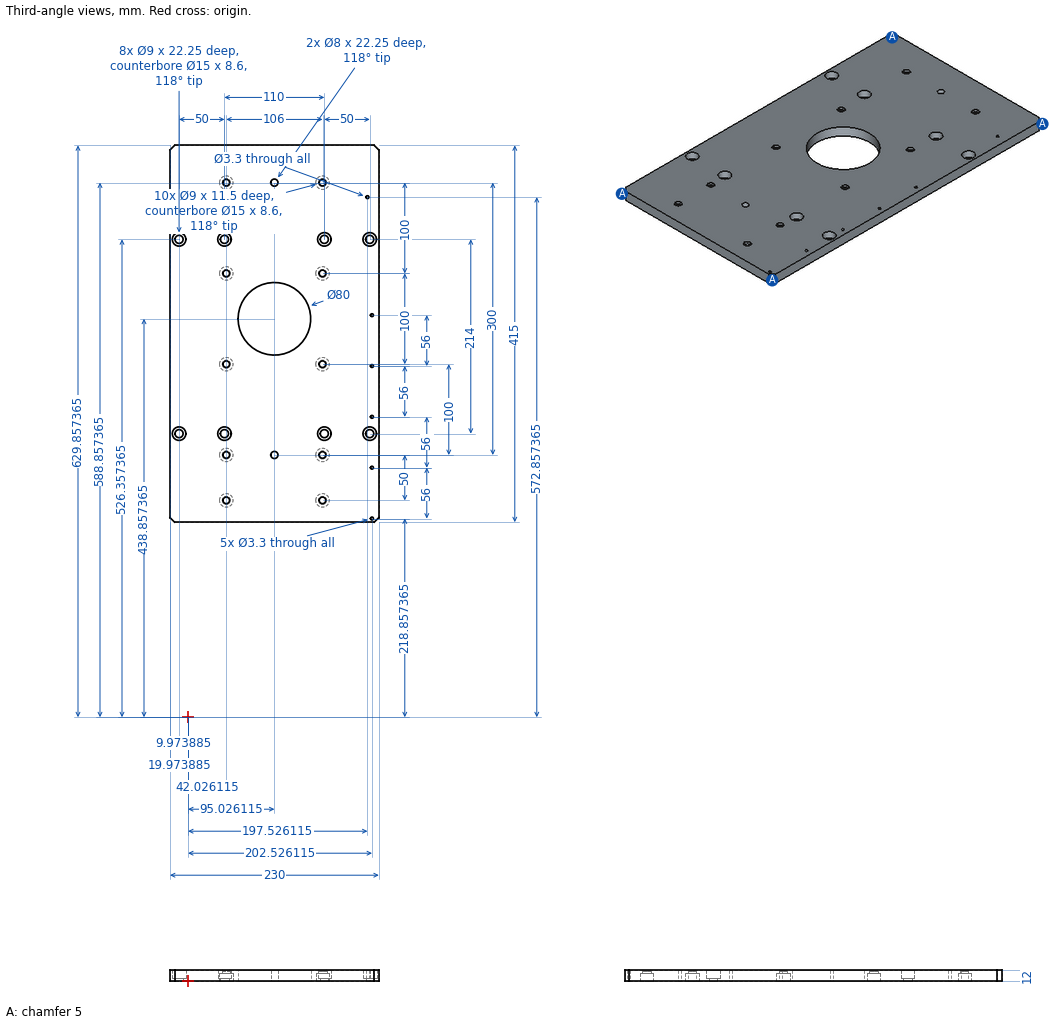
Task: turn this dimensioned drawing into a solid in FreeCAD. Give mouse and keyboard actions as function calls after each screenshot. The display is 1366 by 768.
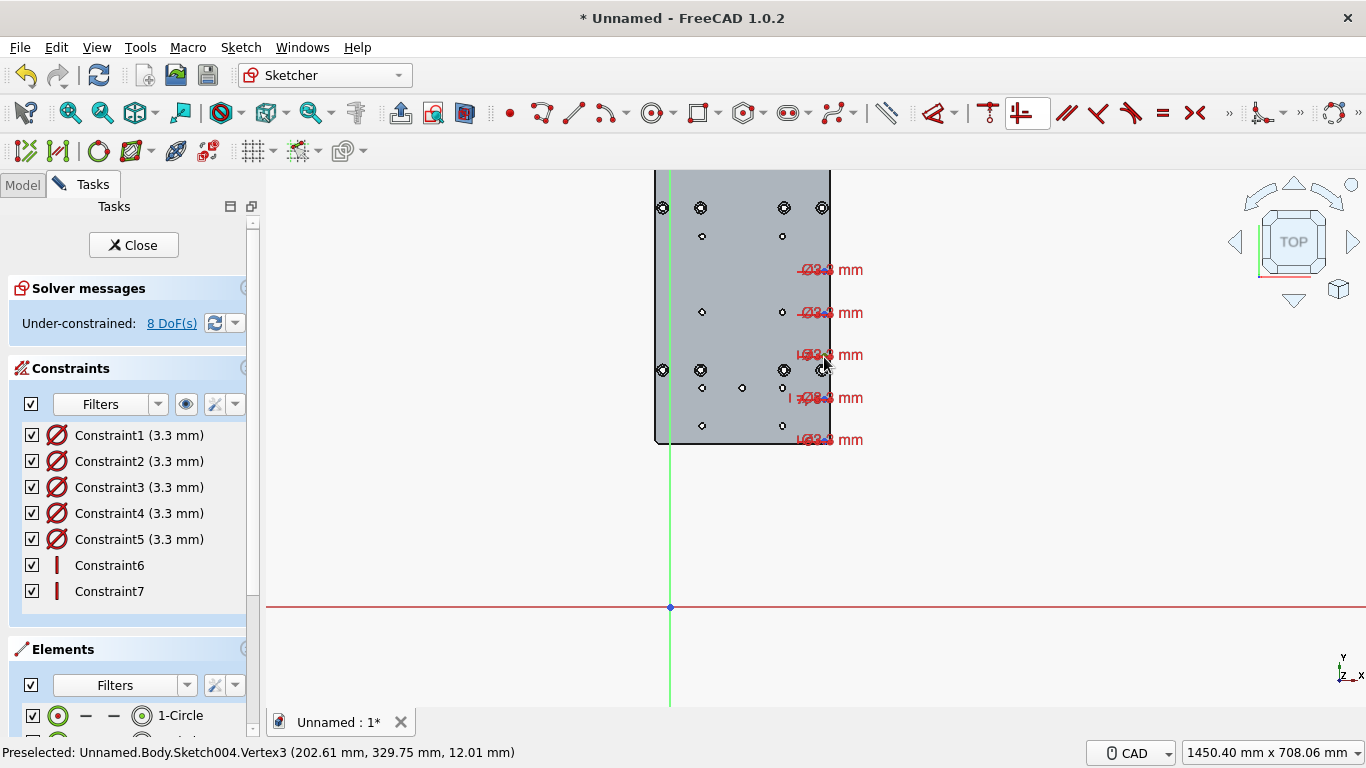
click(824, 315)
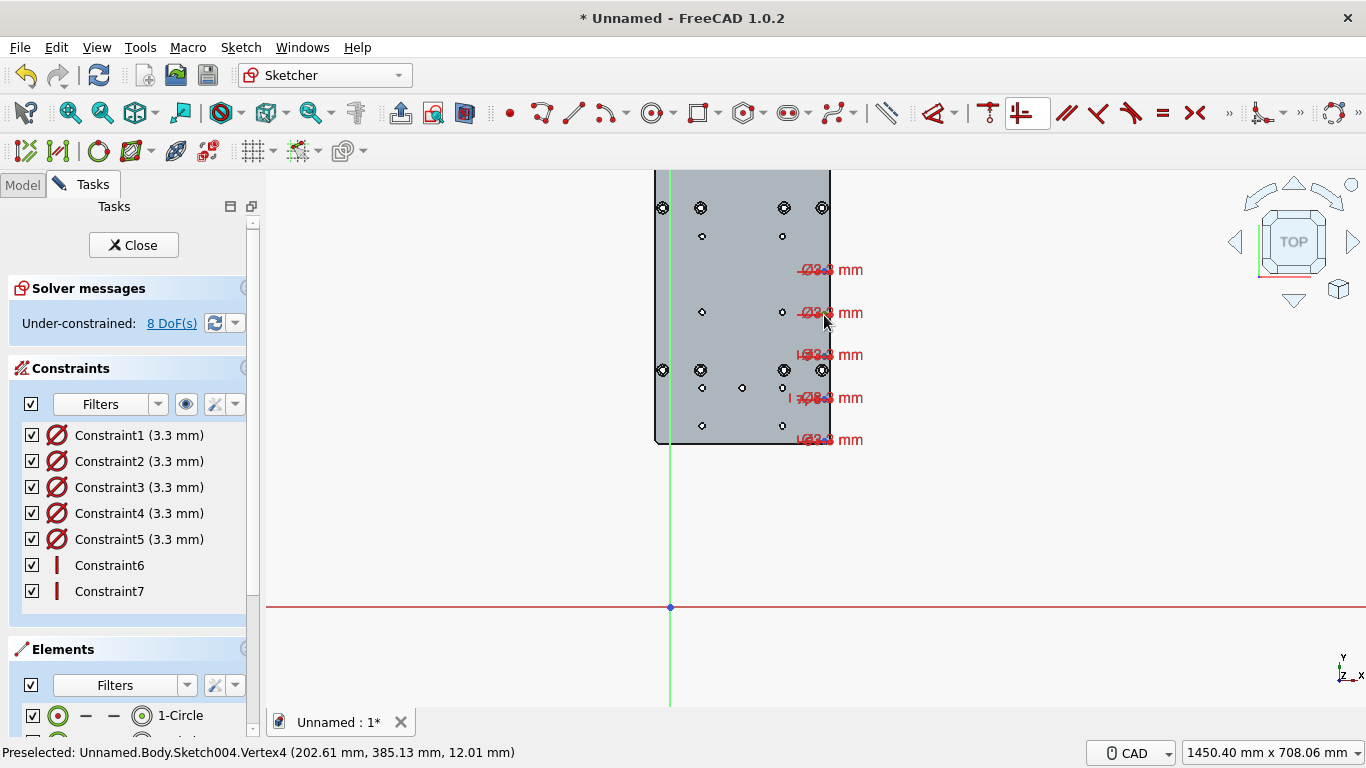
click(1044, 114)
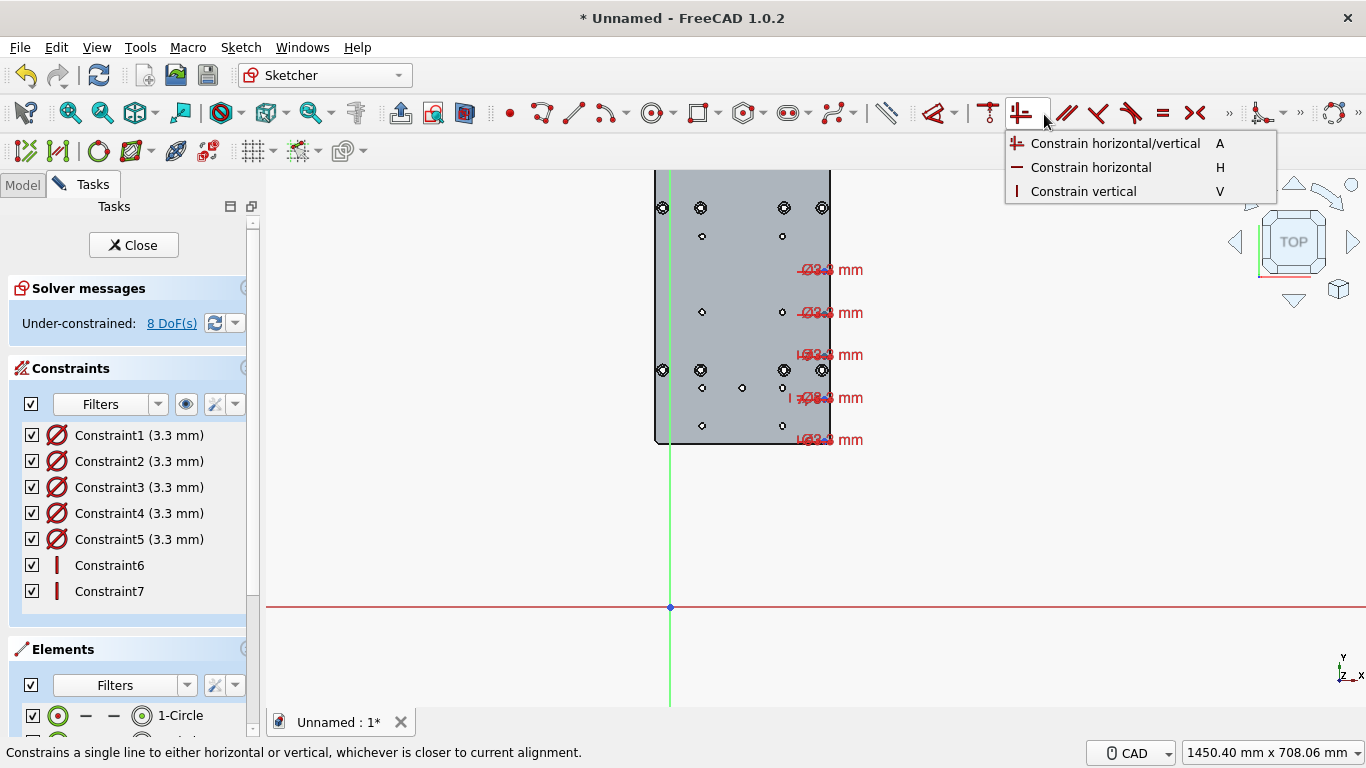
click(1141, 191)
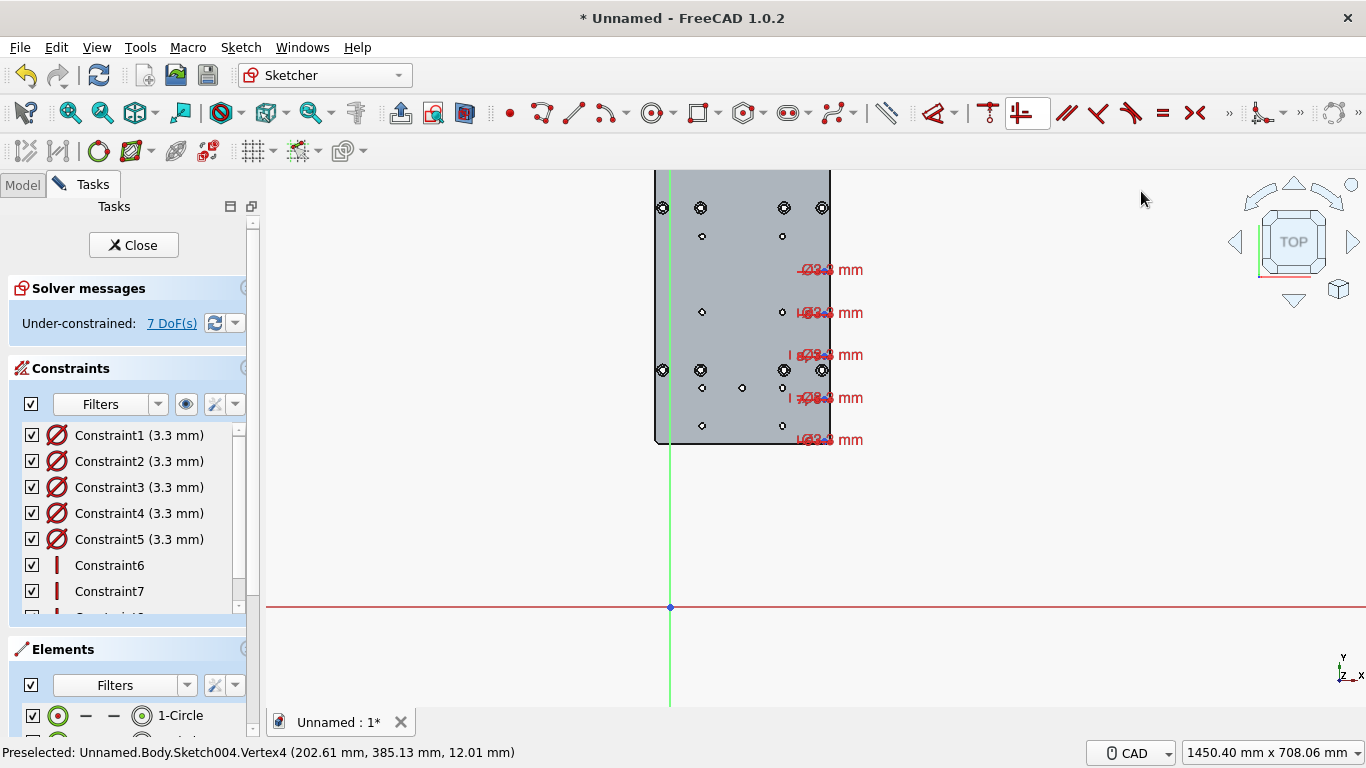
click(824, 315)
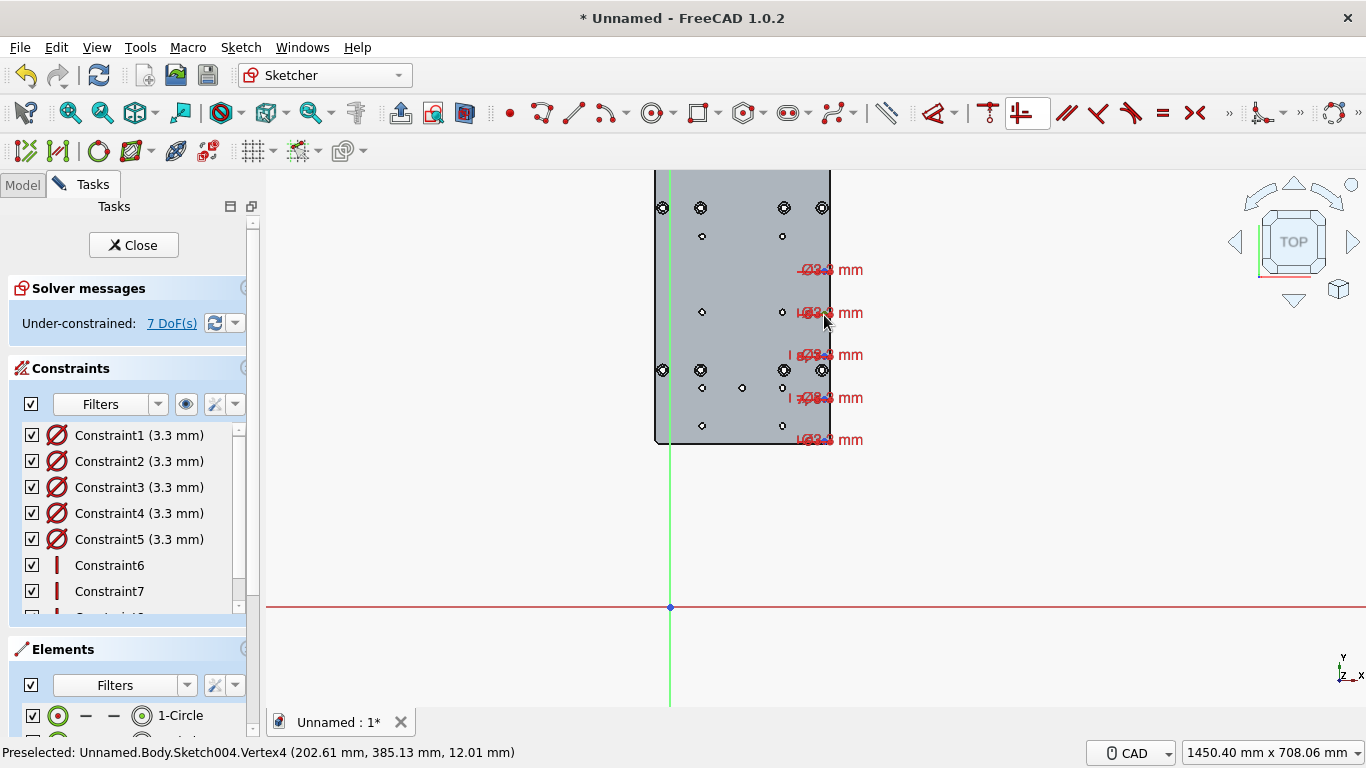
click(824, 272)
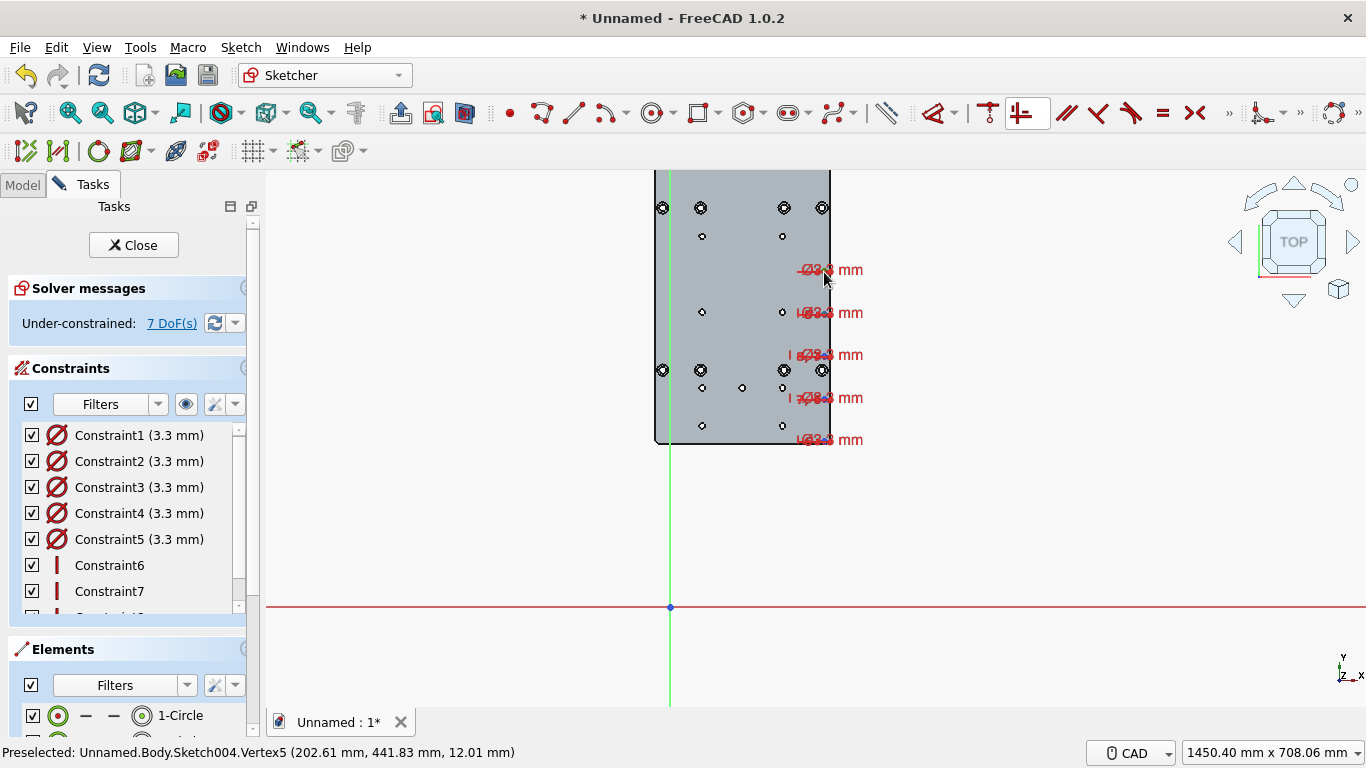
key(v)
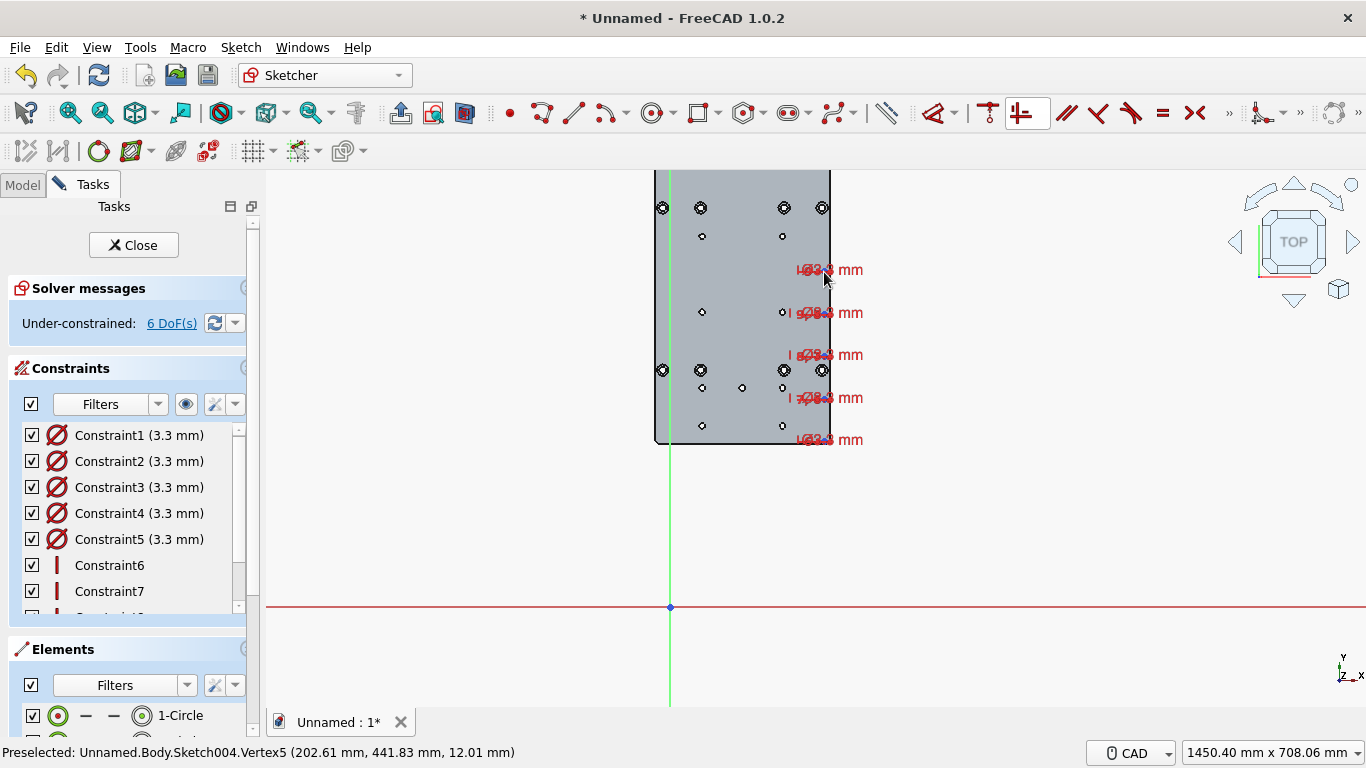
click(934, 114)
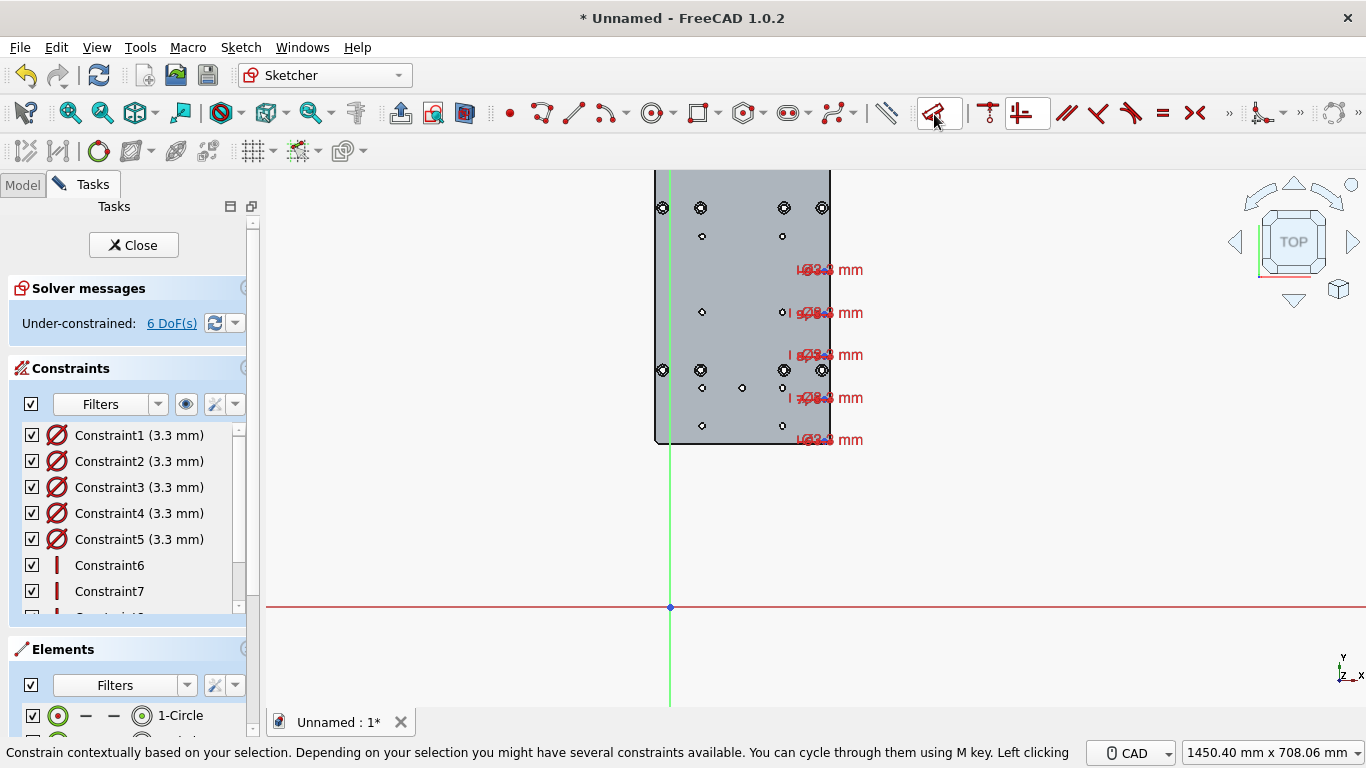
click(824, 442)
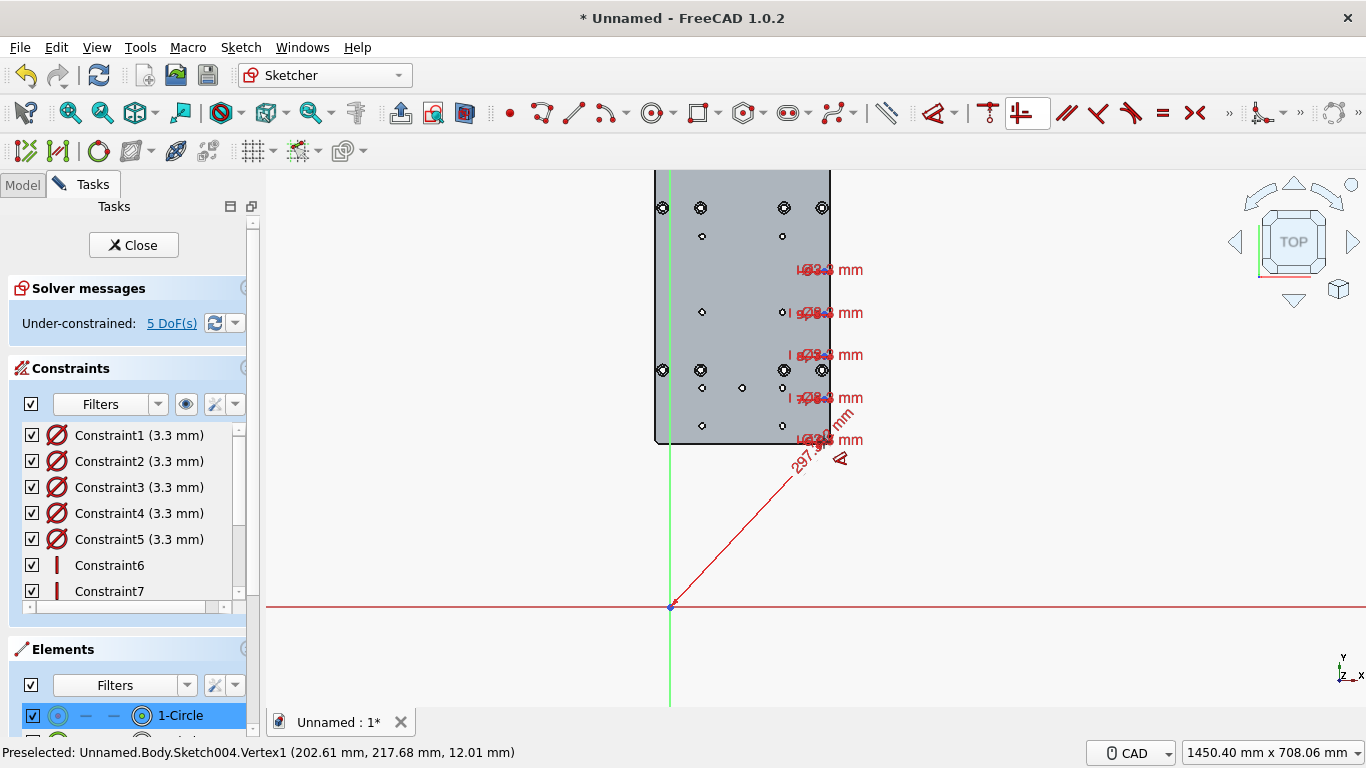
click(824, 400)
click(858, 421)